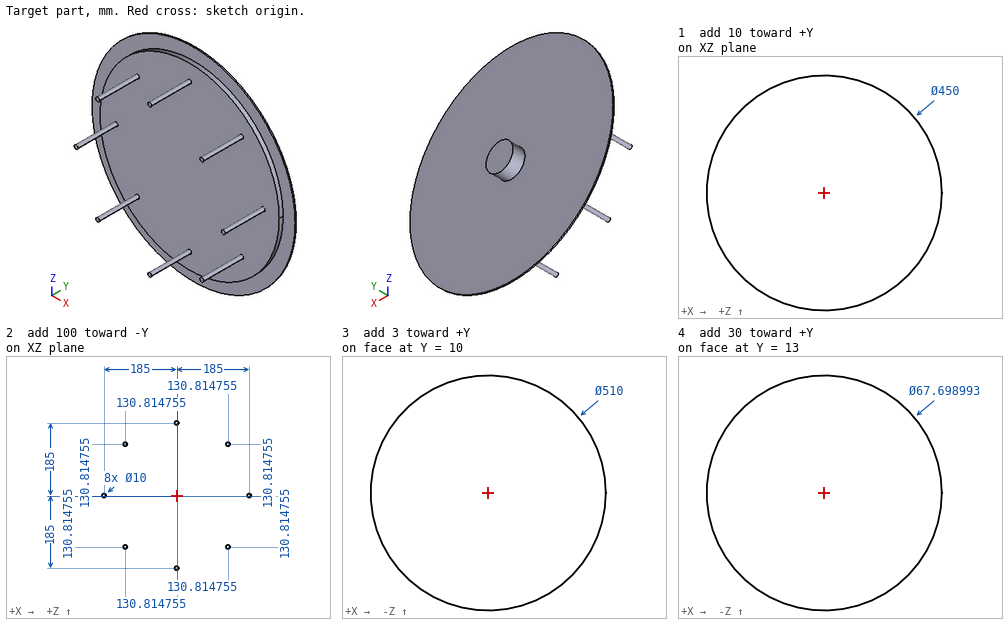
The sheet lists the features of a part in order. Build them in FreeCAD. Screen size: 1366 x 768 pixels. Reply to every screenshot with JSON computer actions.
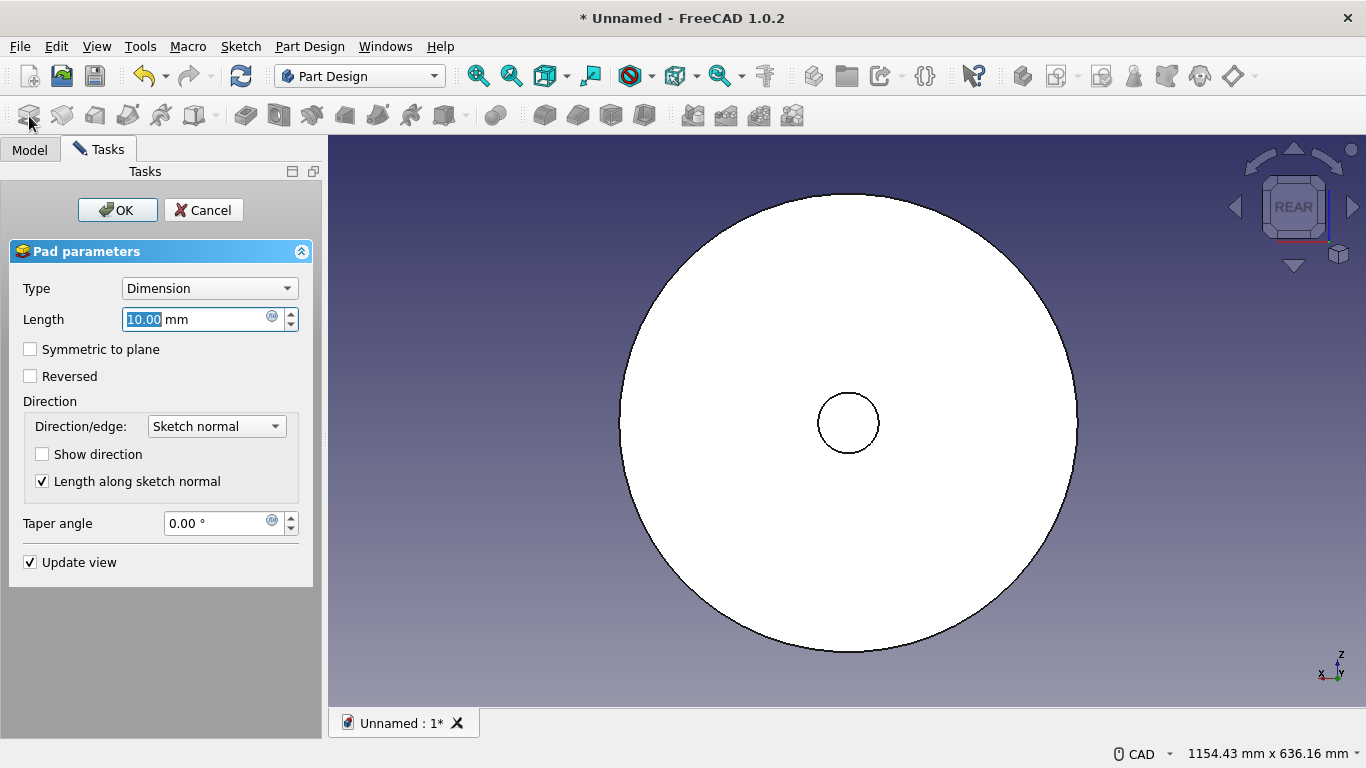
{"action": "type", "text": "30"}
{"action": "key", "text": "Tab"}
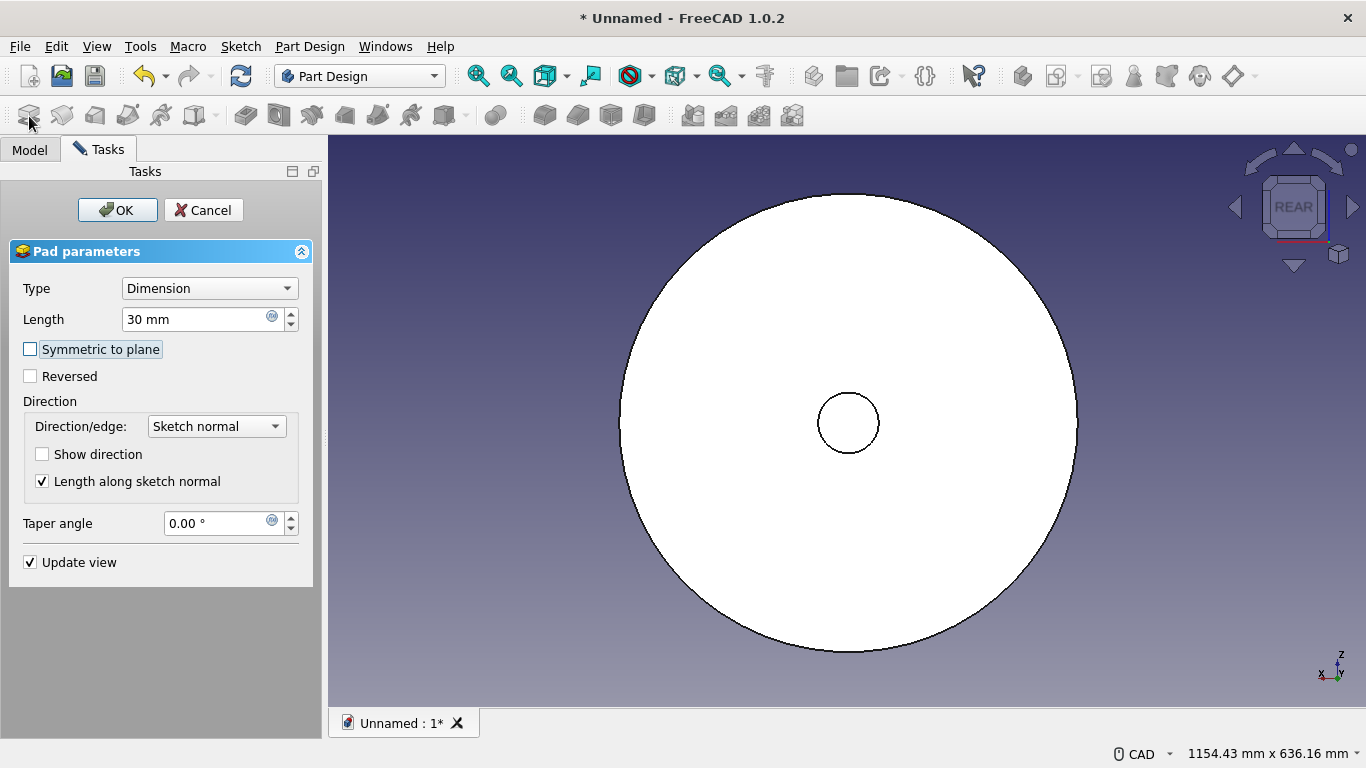
{"action": "left_click", "coordinate": [118, 210]}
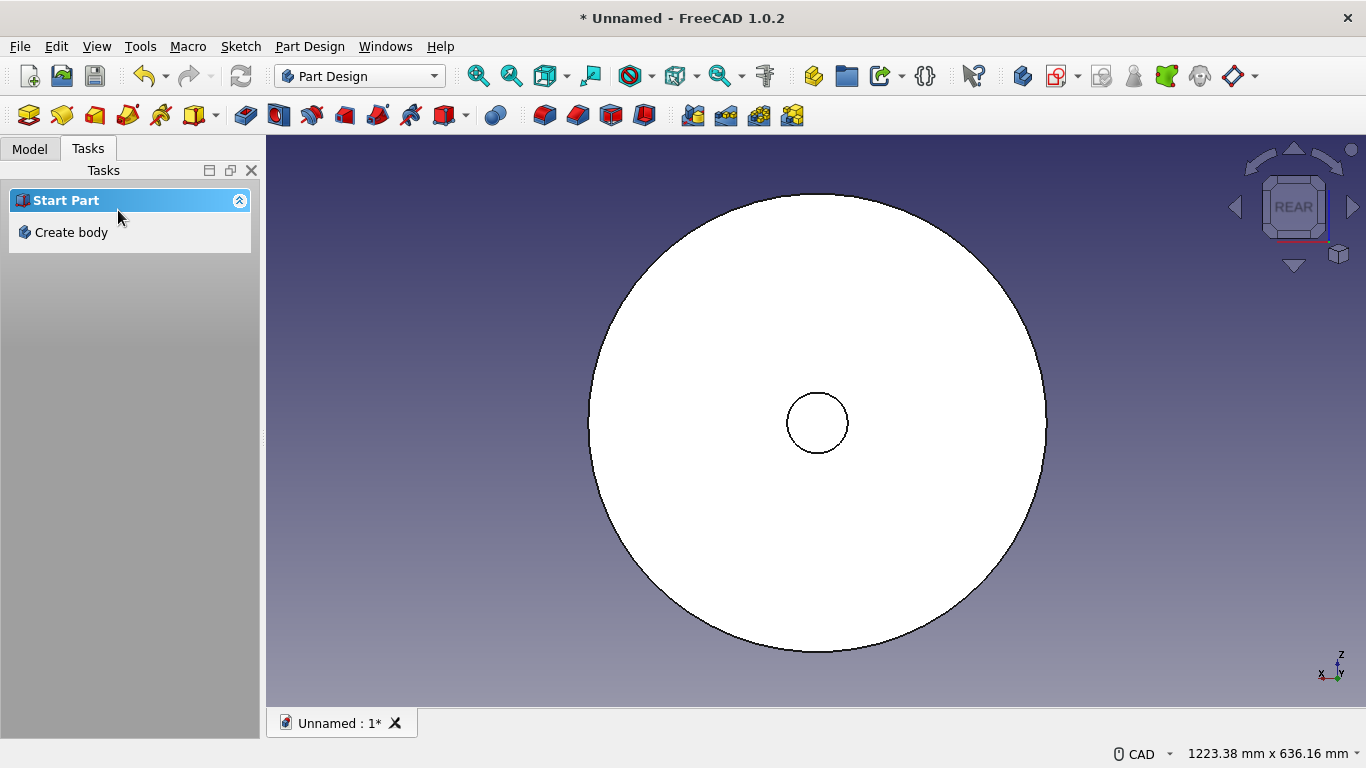
{"action": "key", "text": "0"}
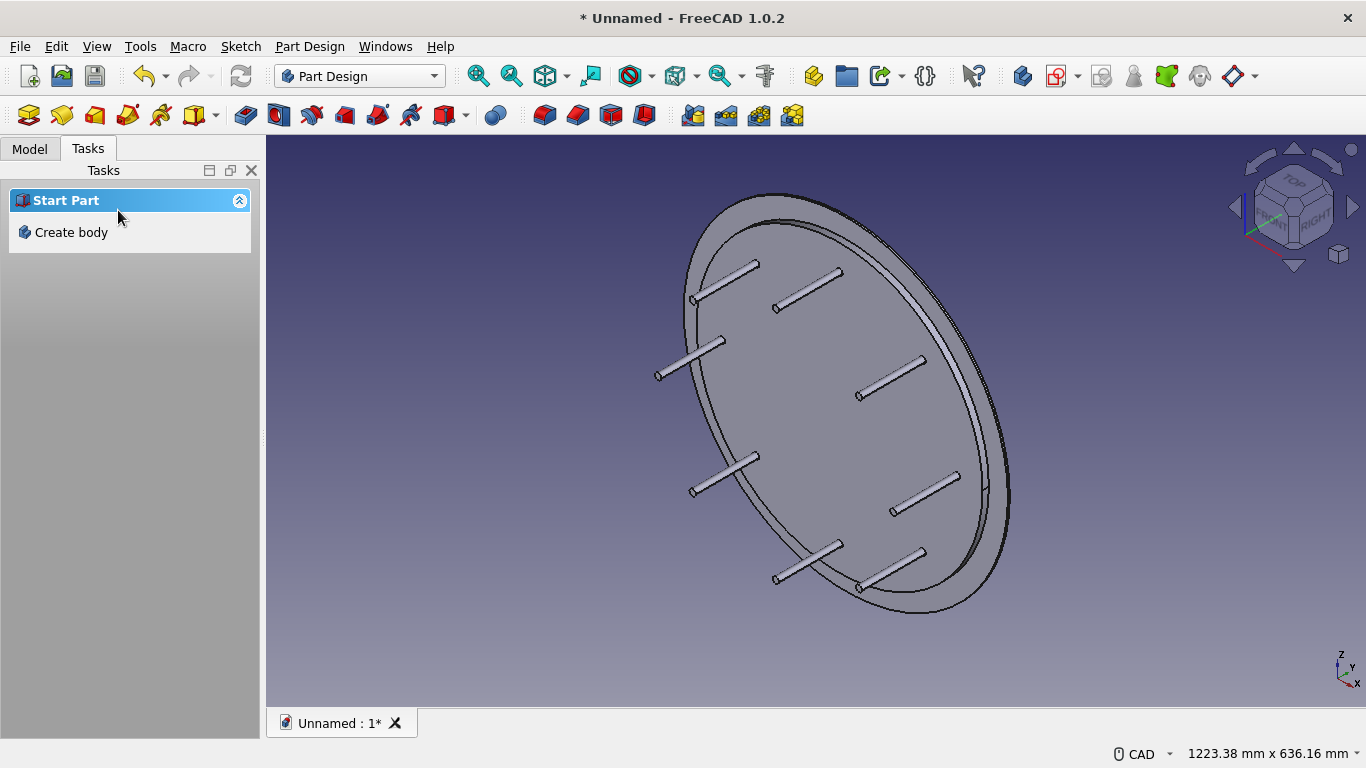
{"action": "left_click", "coordinate": [479, 76]}